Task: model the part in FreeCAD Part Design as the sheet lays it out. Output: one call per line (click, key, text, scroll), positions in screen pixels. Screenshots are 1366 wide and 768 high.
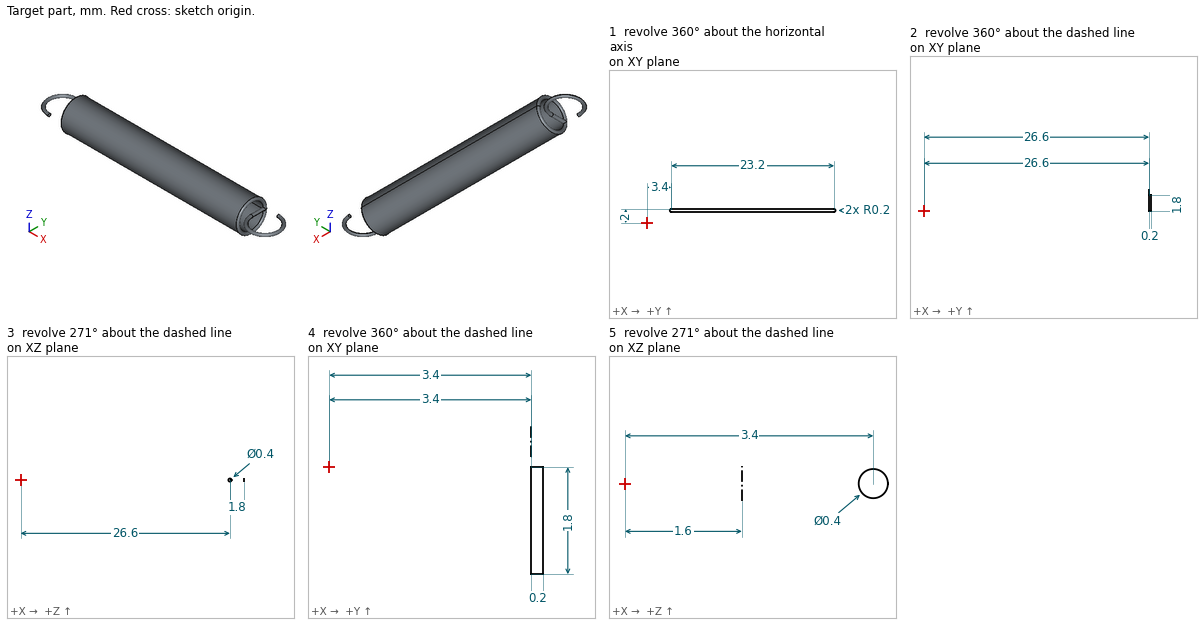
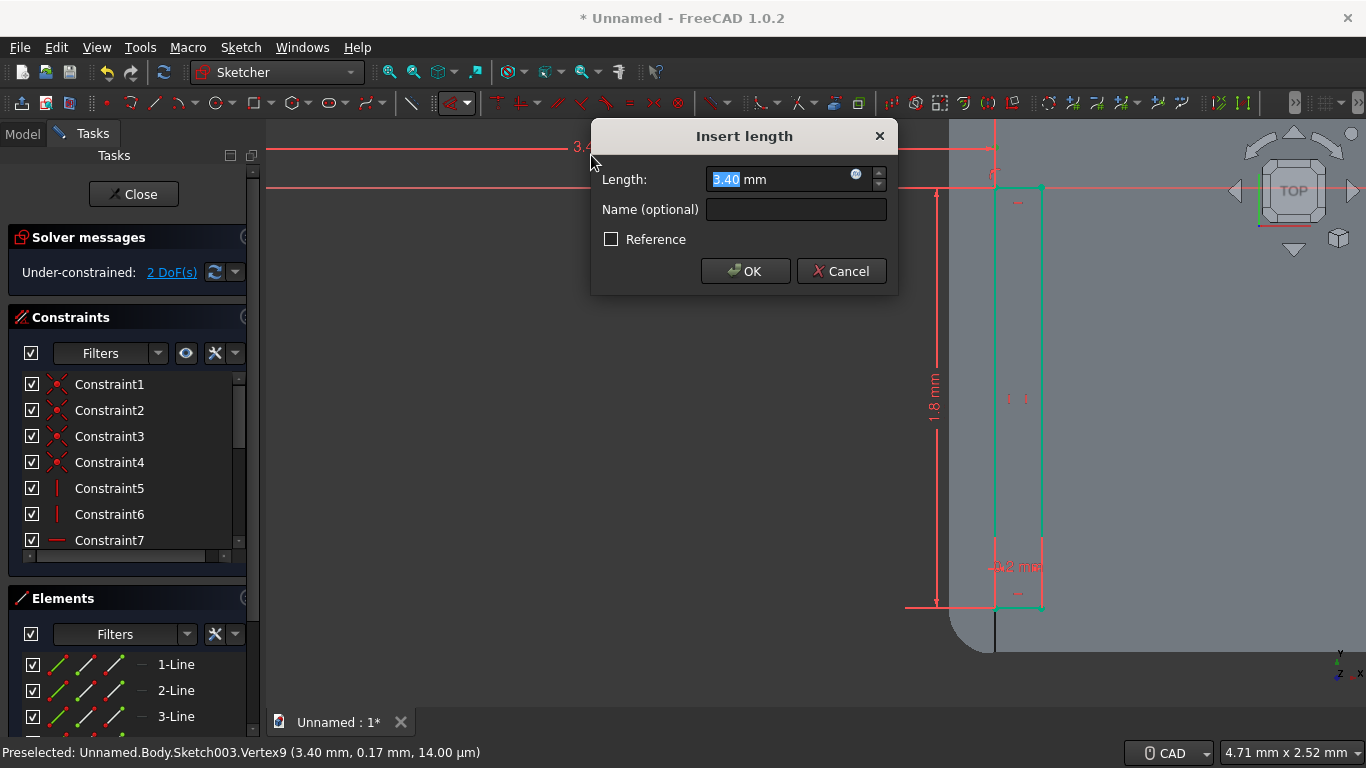
text(3.4)
key(Return)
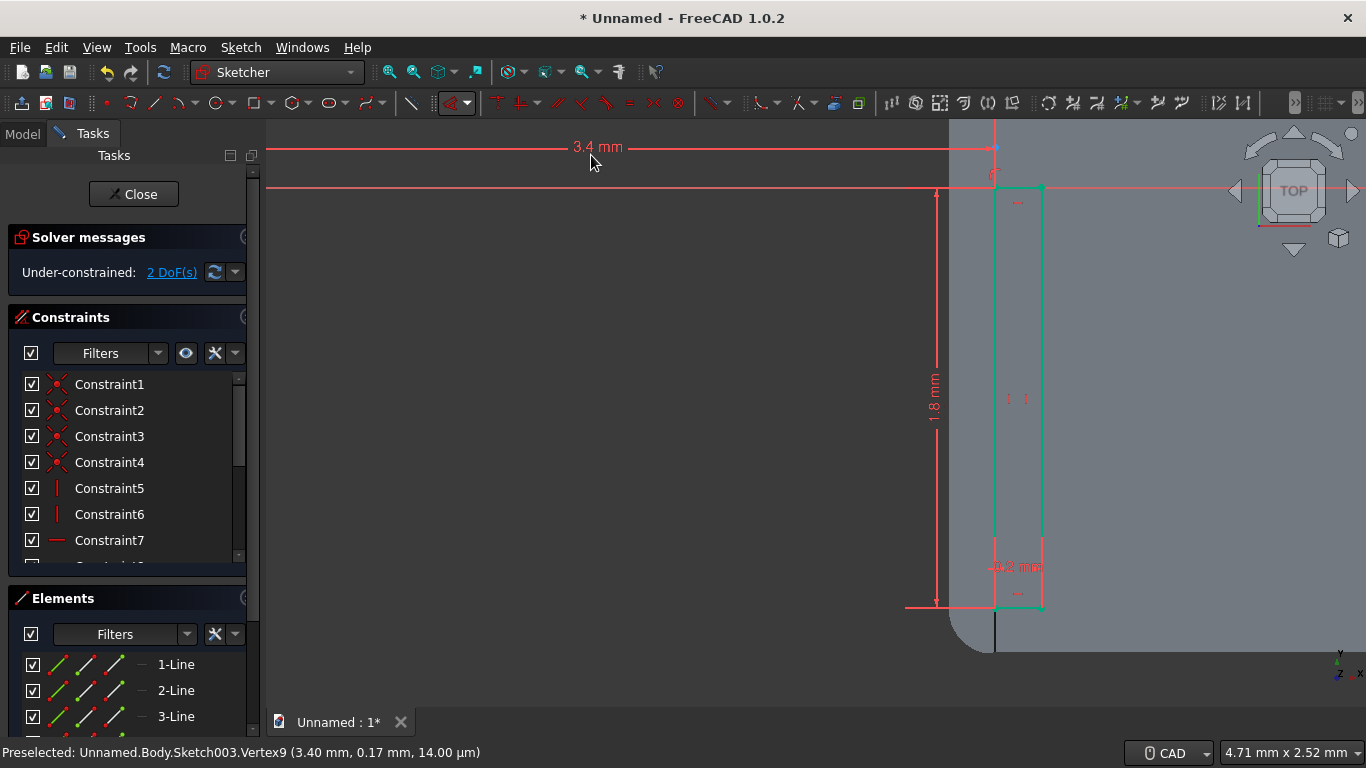
click(134, 194)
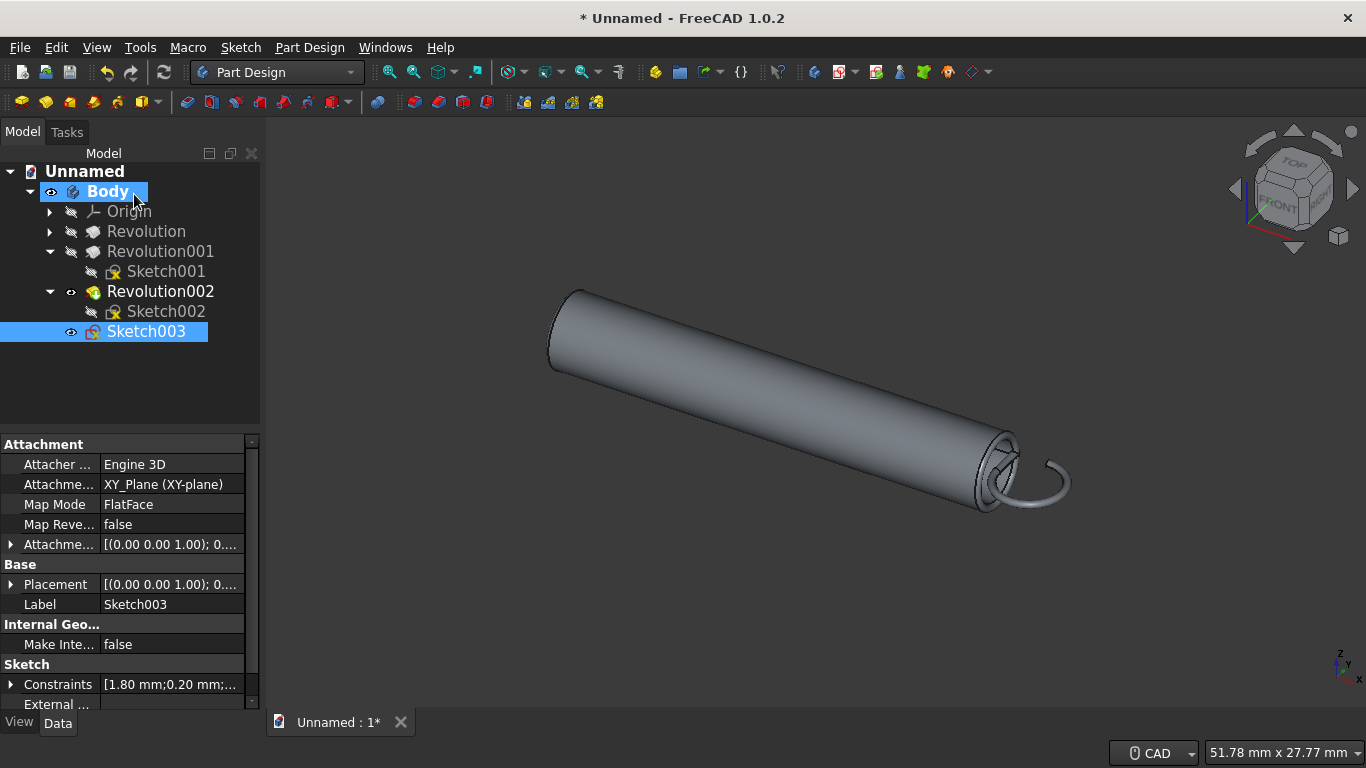
click(46, 102)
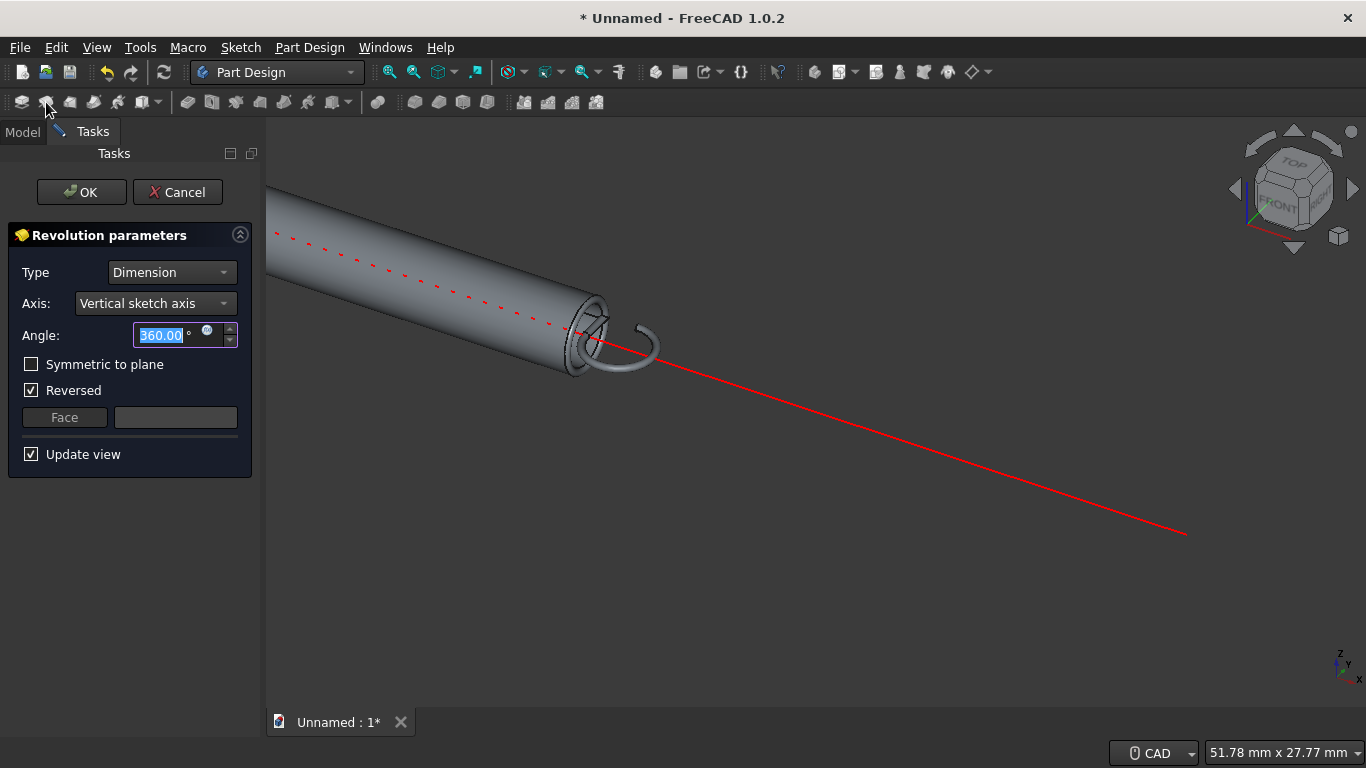
click(156, 304)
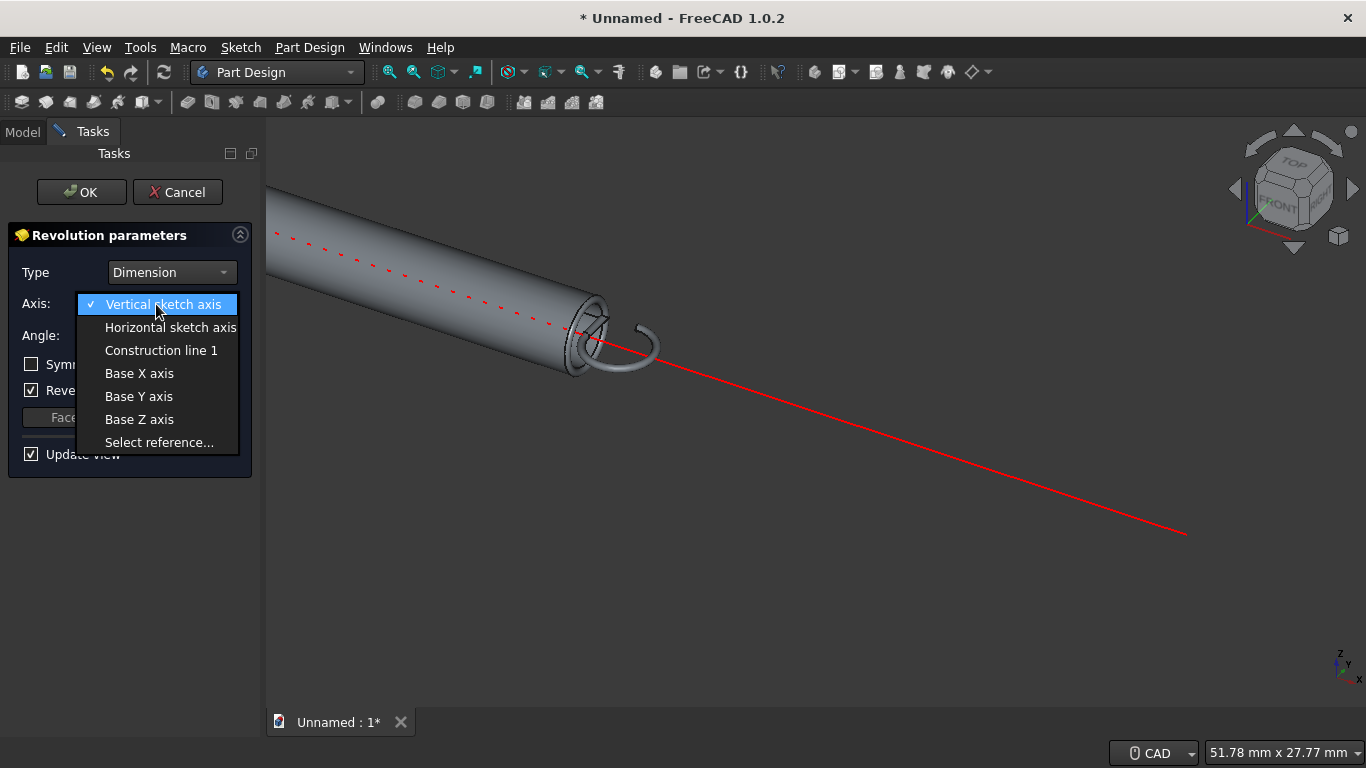
click(156, 350)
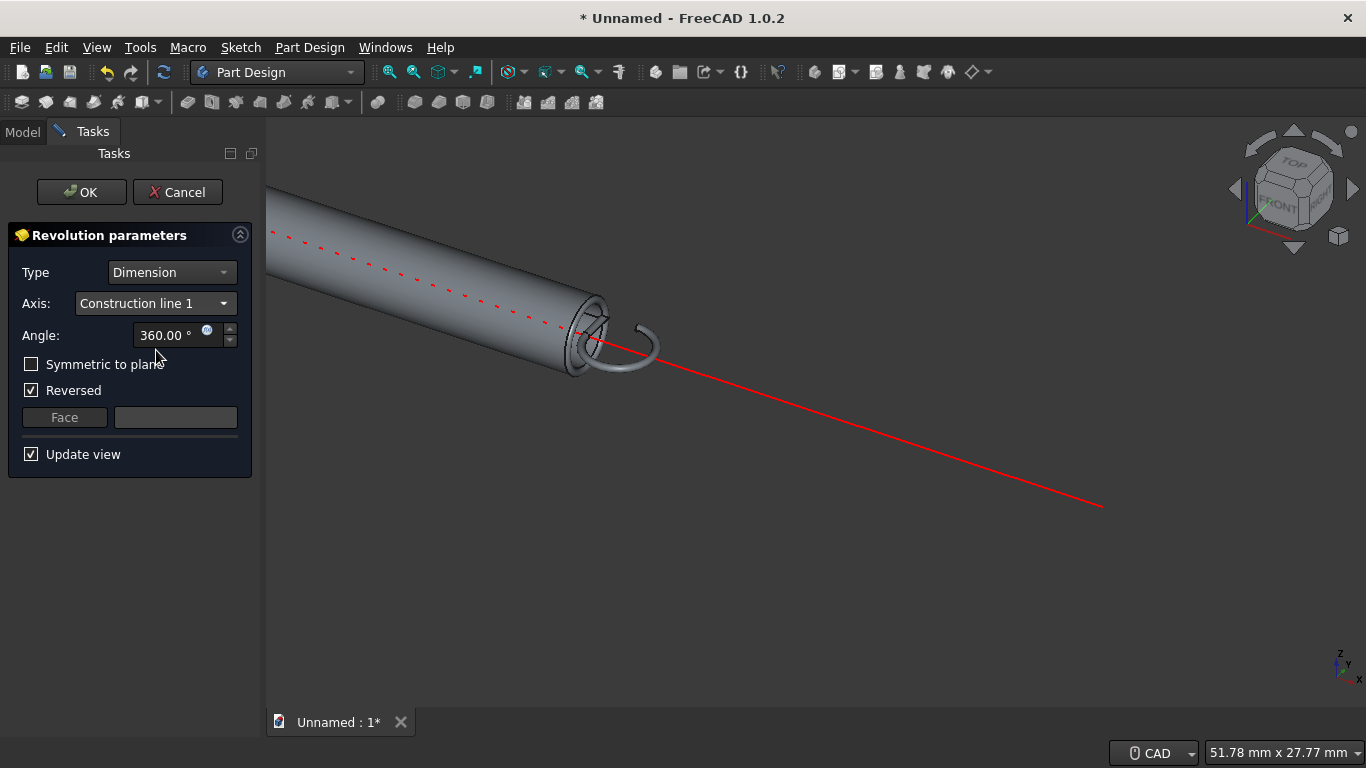
click(82, 192)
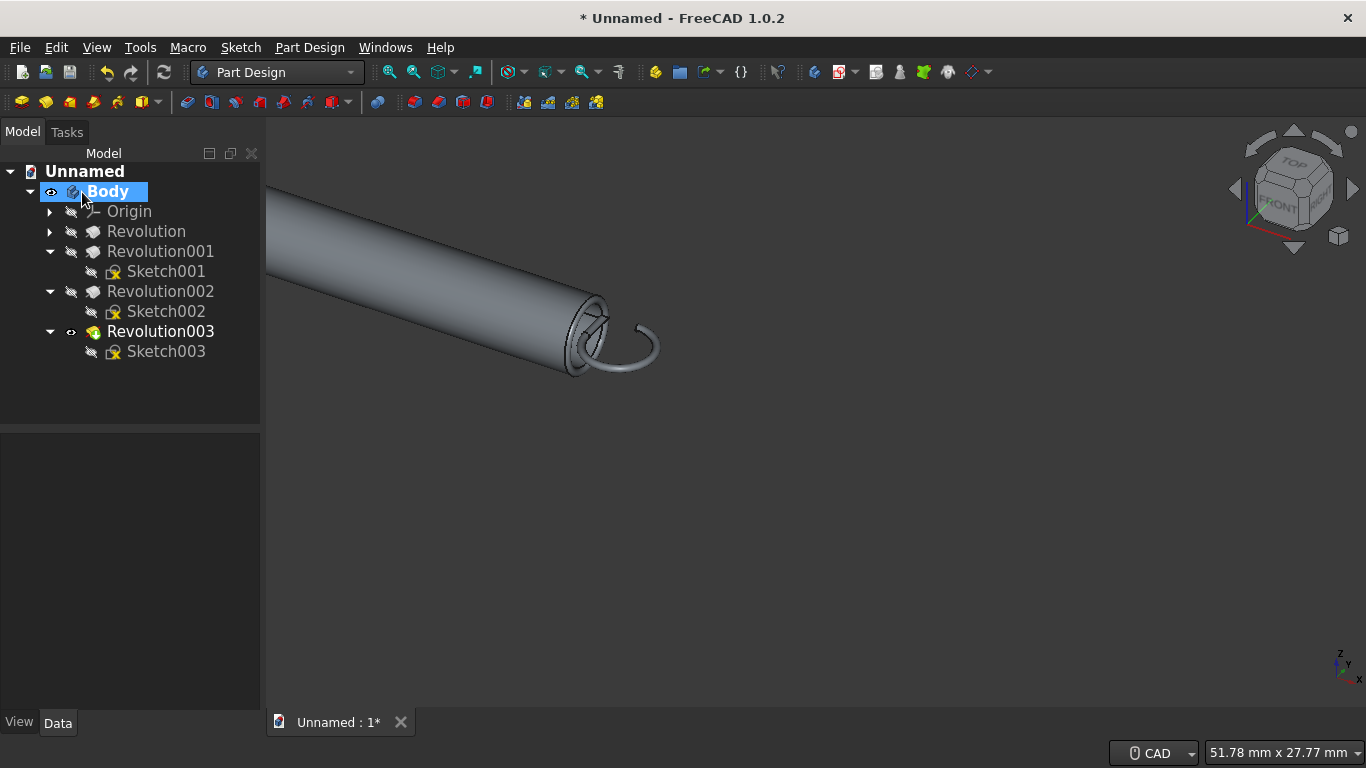
key(v)
key(f)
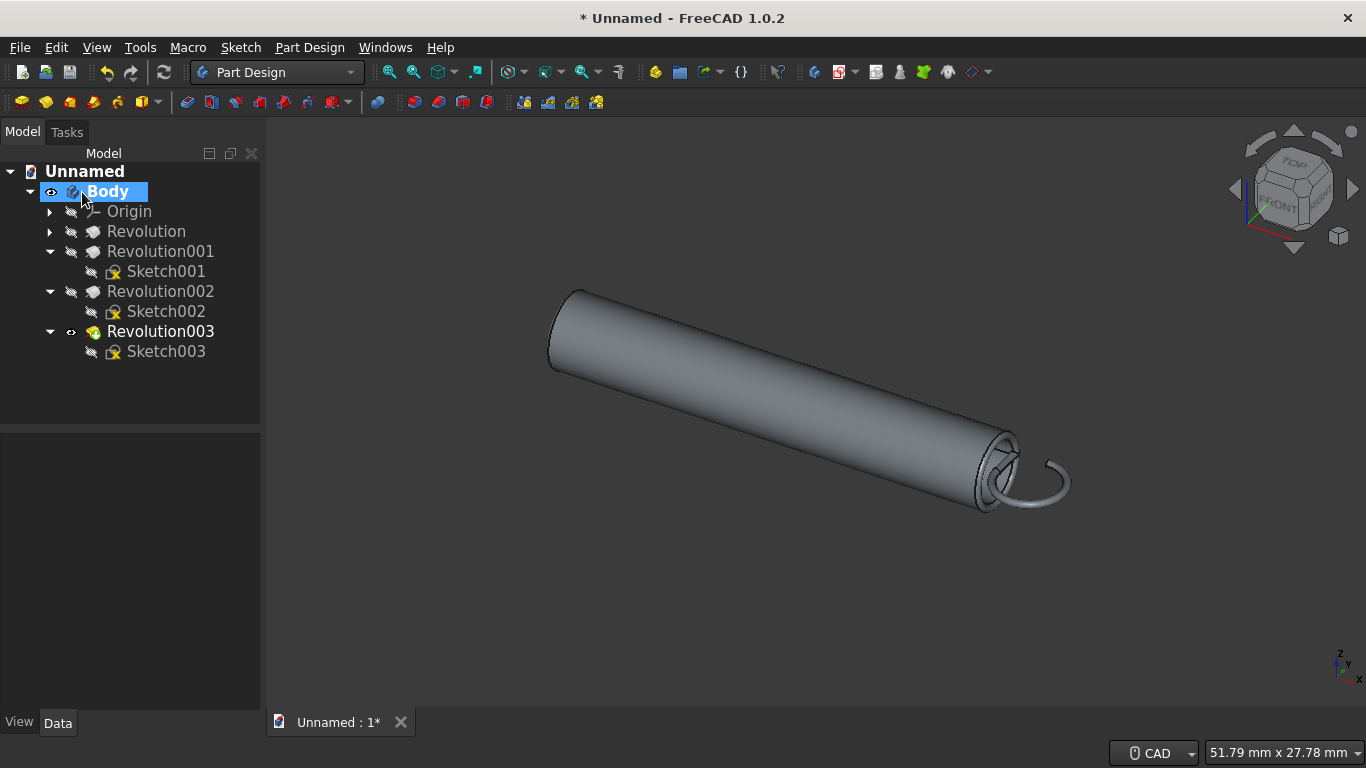
click(840, 72)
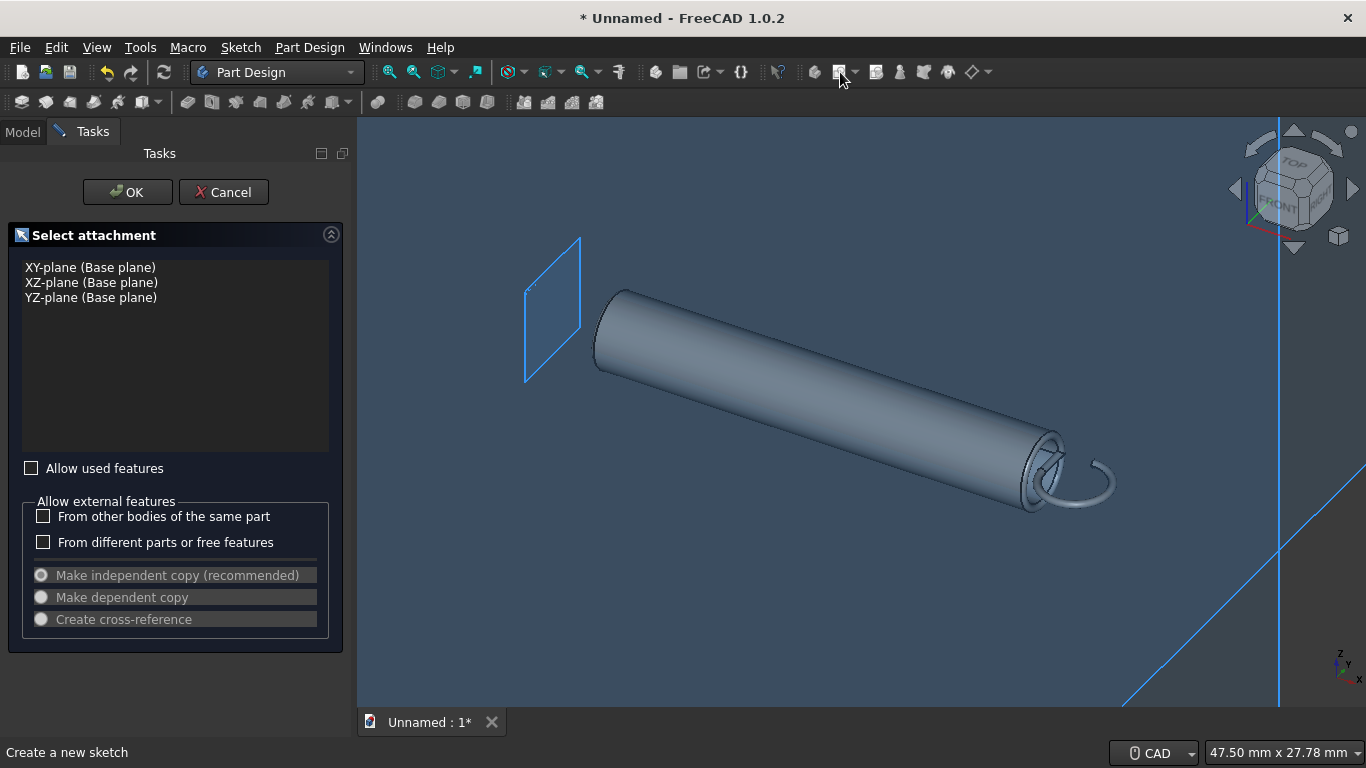
click(82, 282)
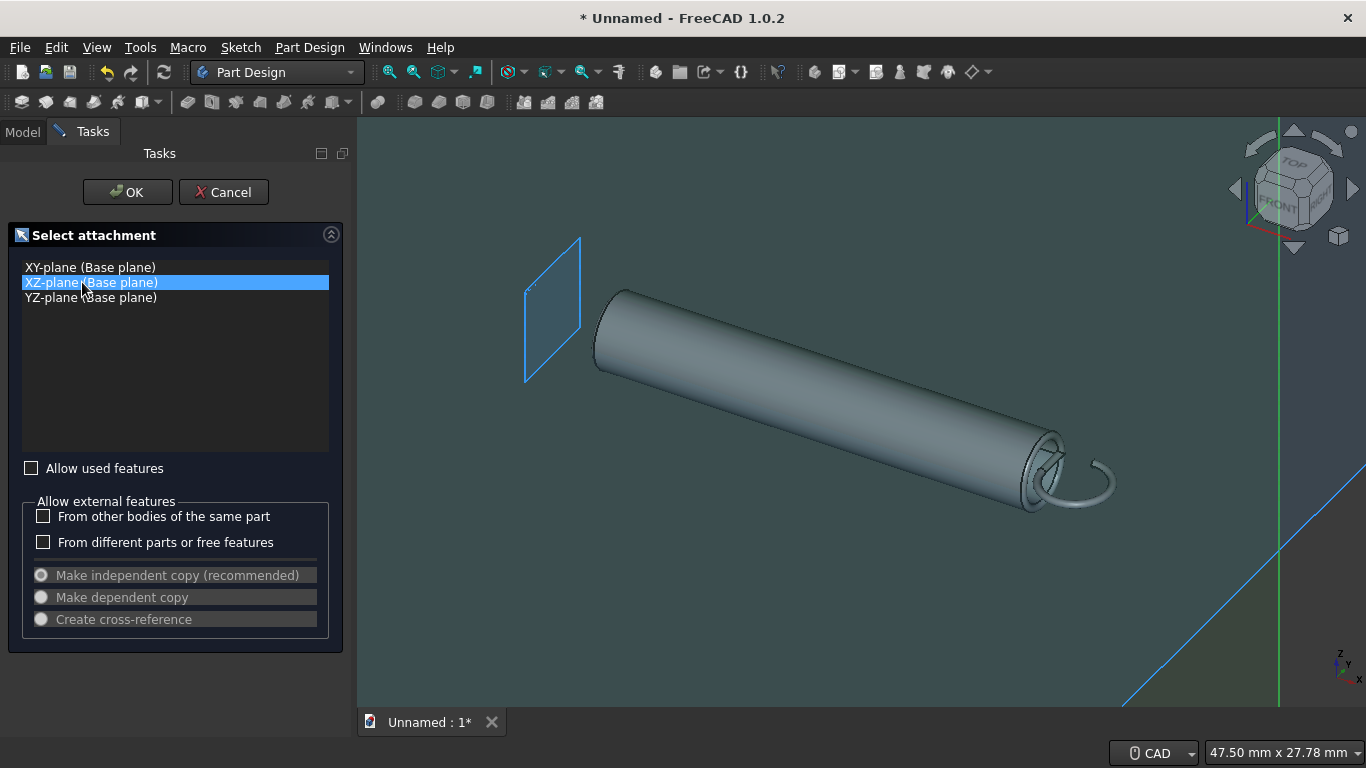
click(128, 192)